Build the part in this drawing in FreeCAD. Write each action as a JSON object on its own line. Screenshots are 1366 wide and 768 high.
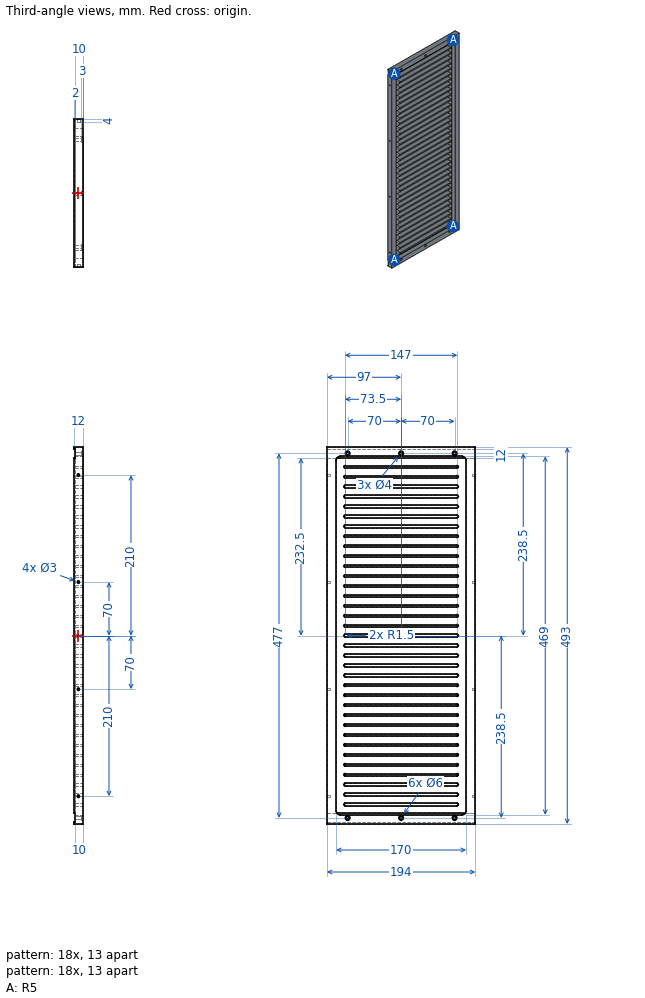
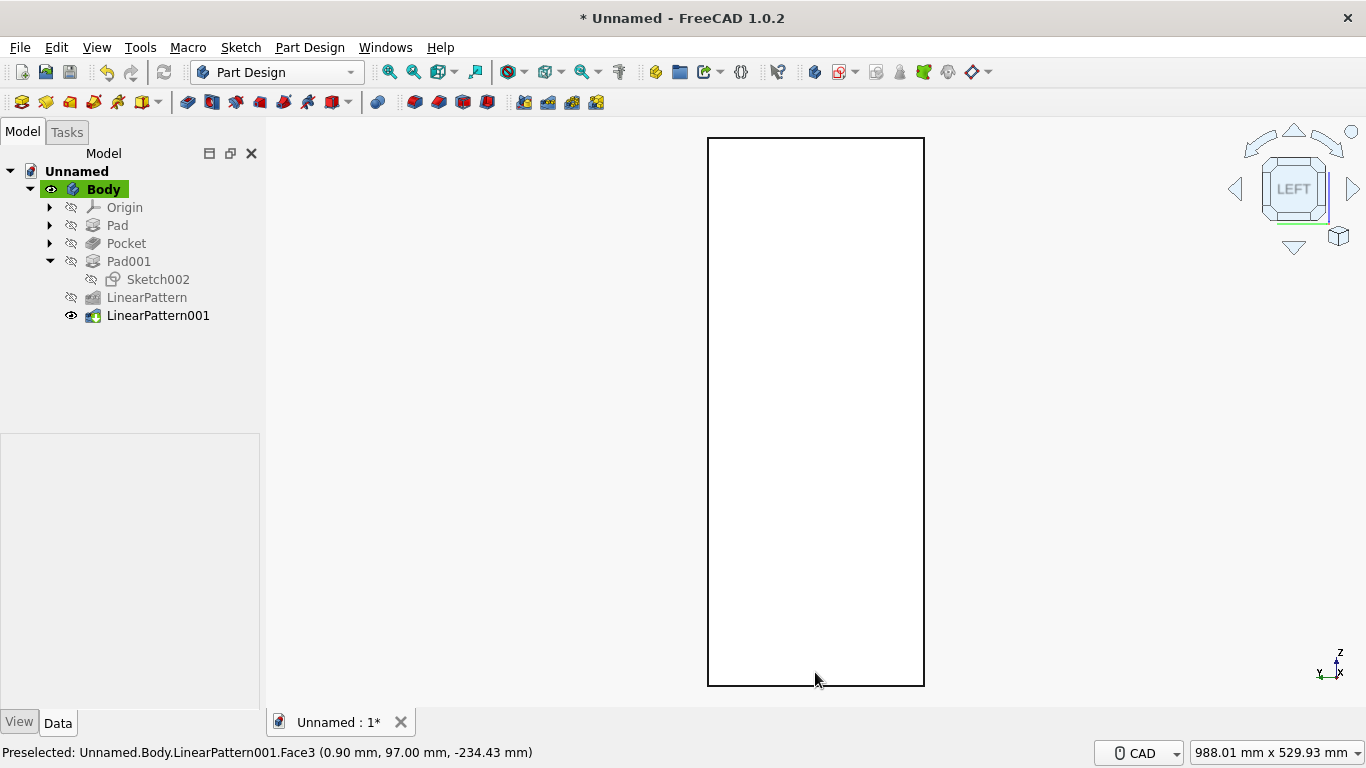
{"action": "scroll", "coordinate": [911, 672], "scroll_direction": "up", "scroll_amount": 7}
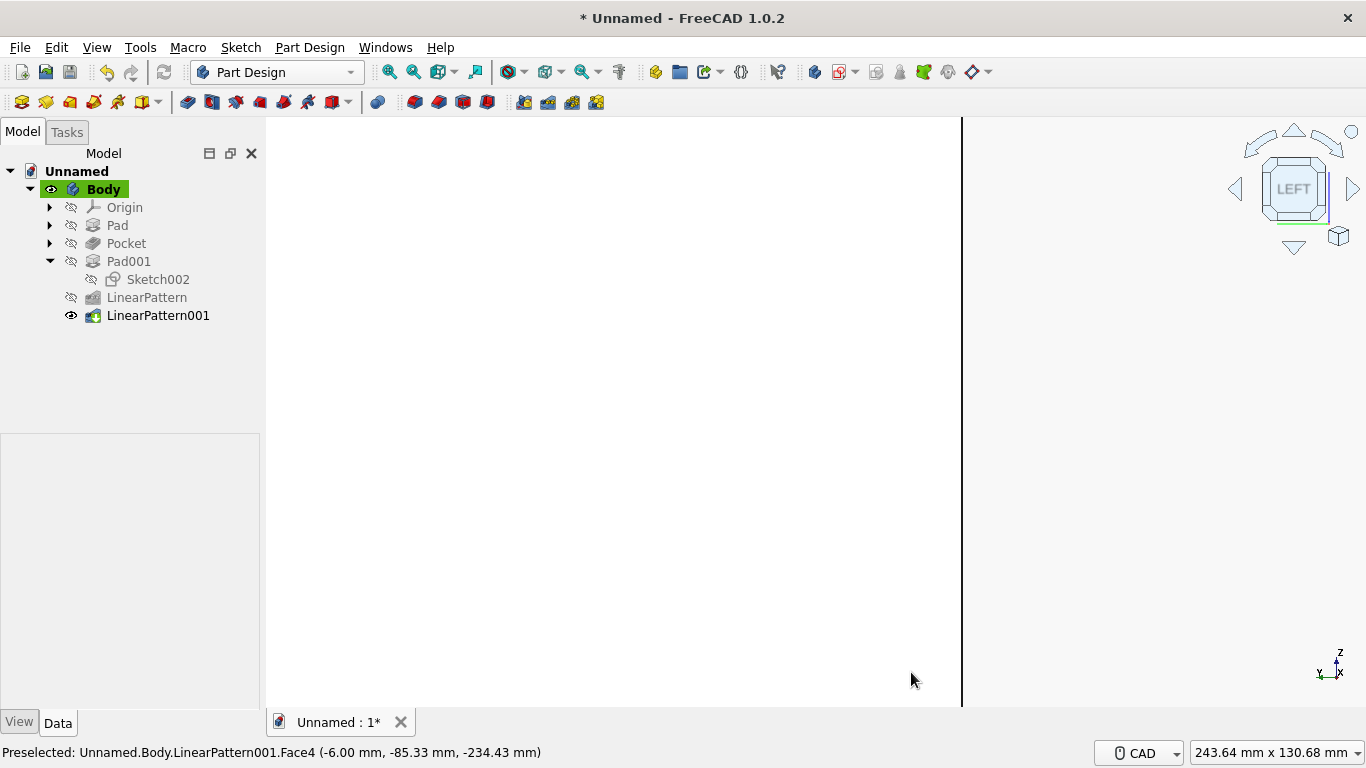
{"action": "key", "text": "v f"}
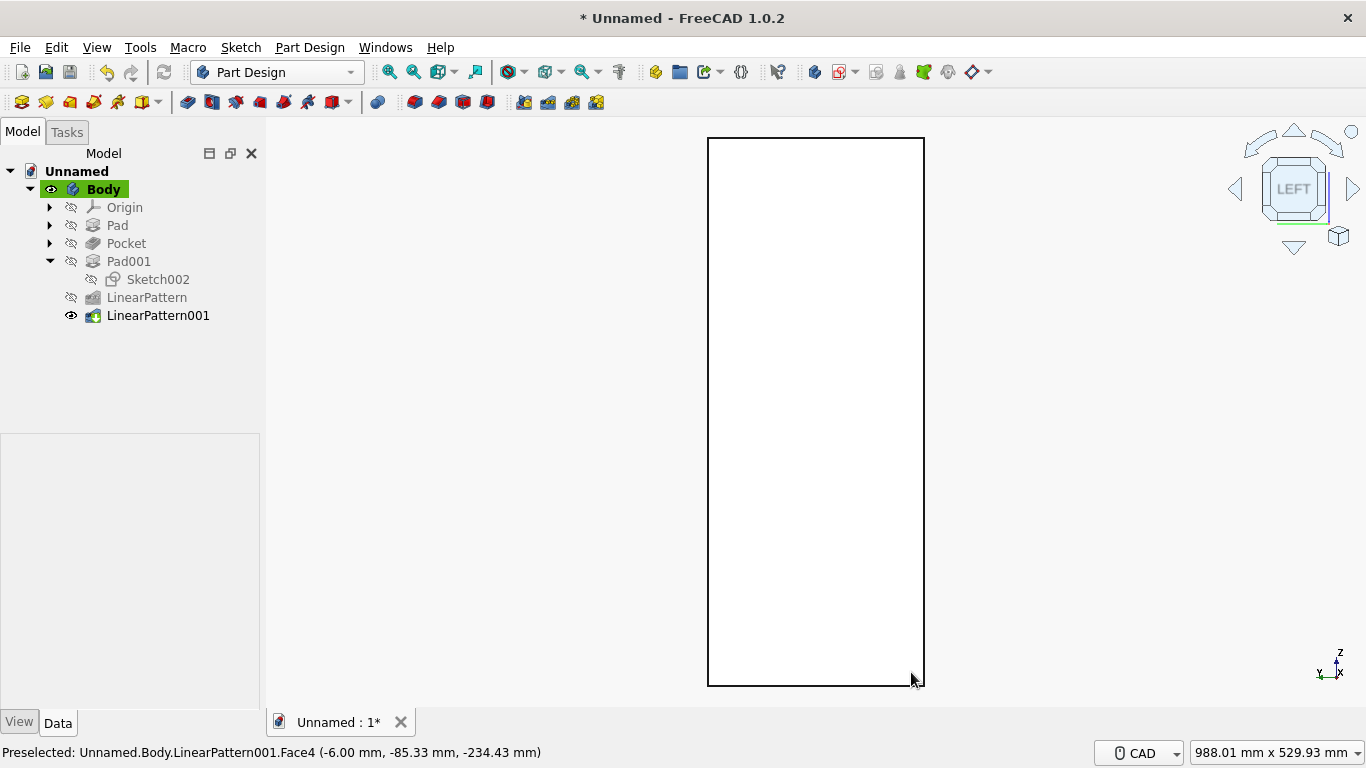
{"action": "key", "text": "v 3"}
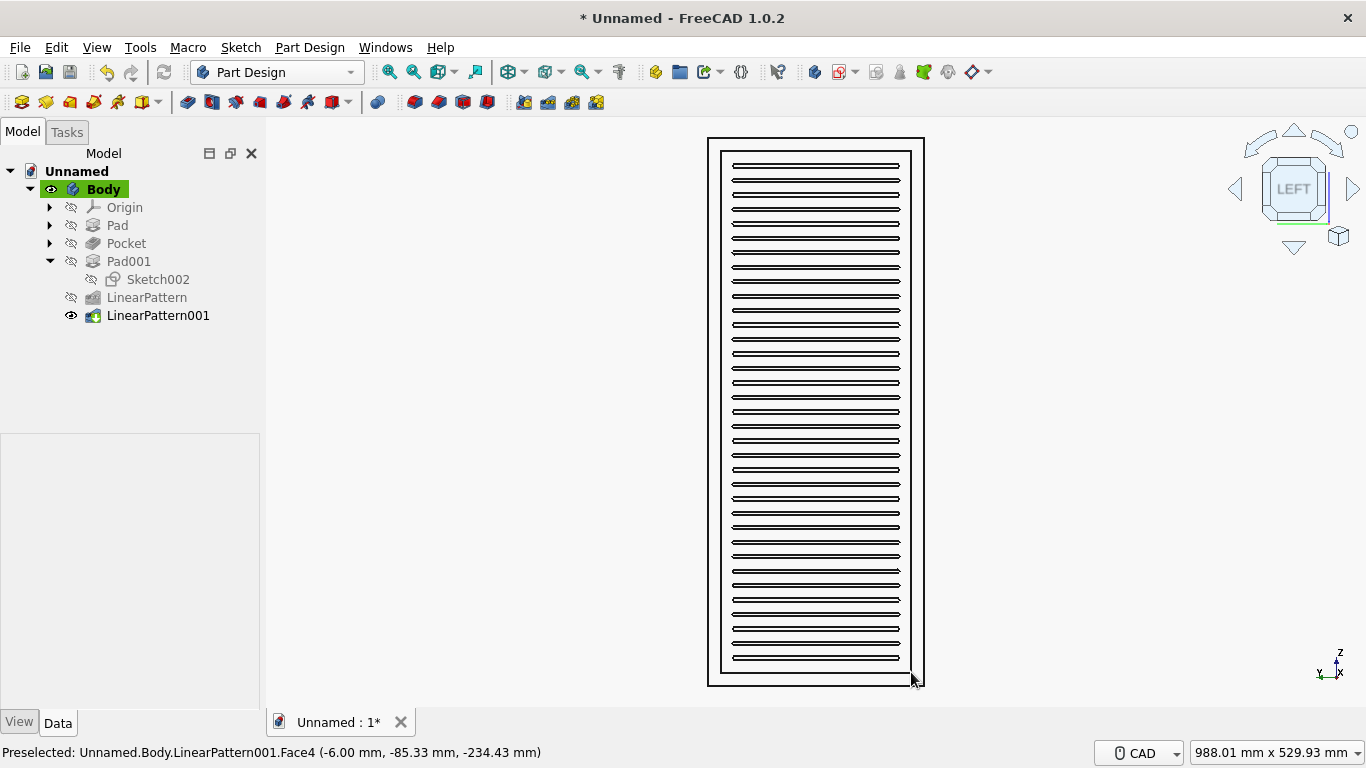
{"action": "key", "text": "0"}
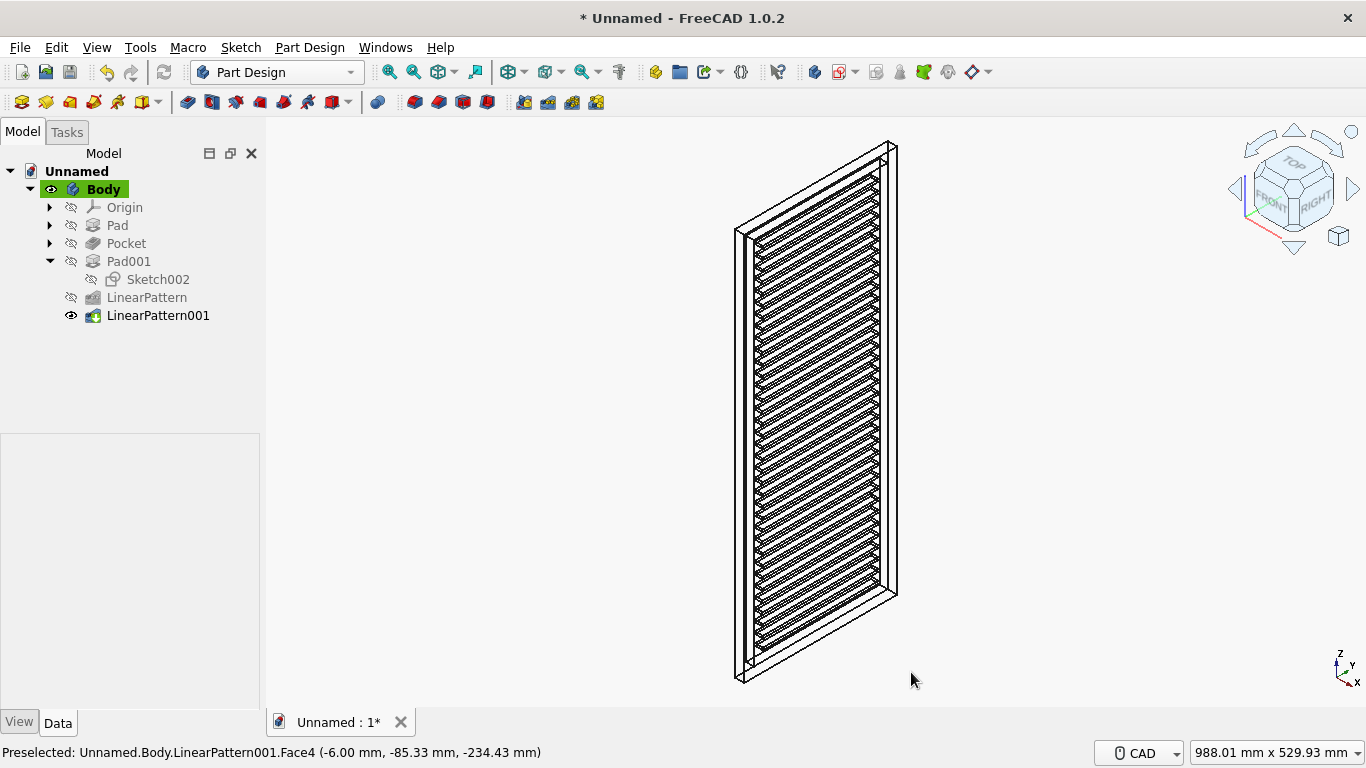
{"action": "scroll", "coordinate": [750, 663], "scroll_direction": "up", "scroll_amount": 7}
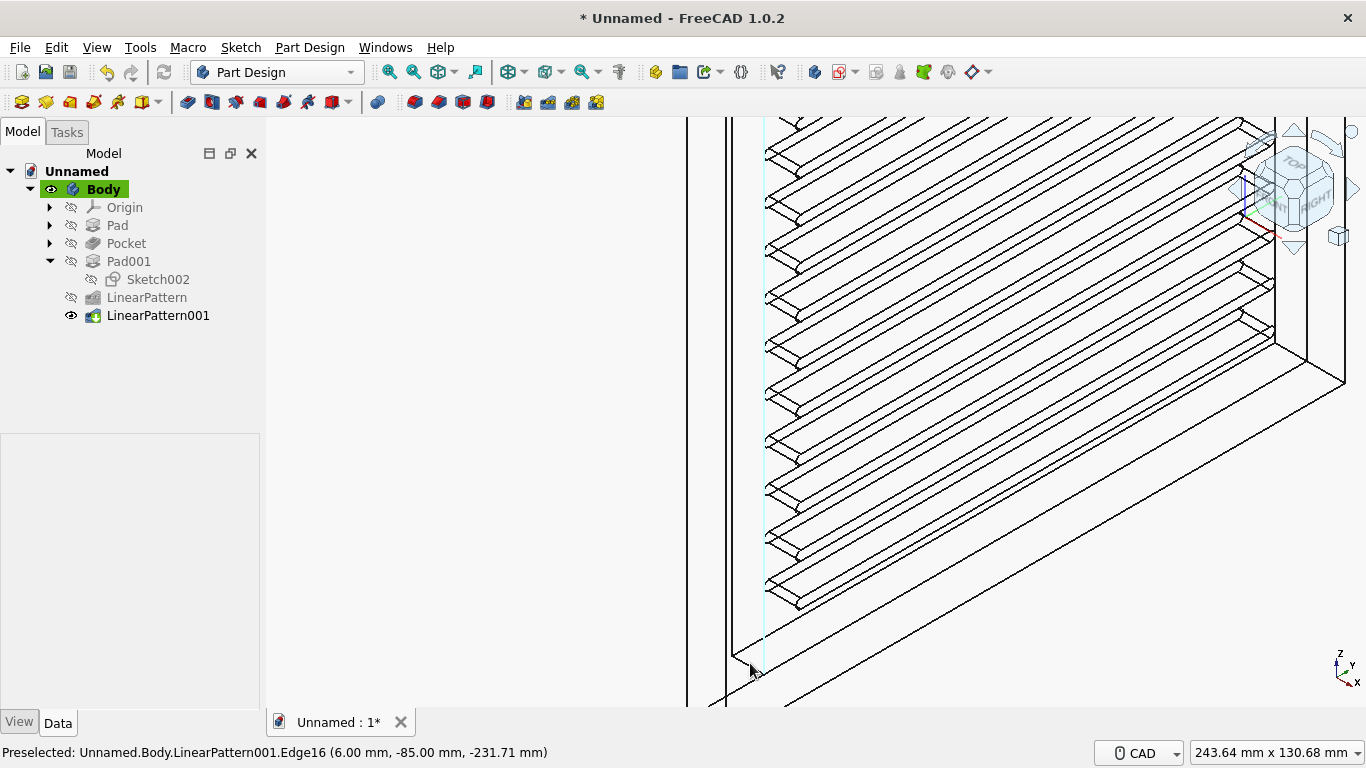
{"action": "left_click", "coordinate": [748, 664]}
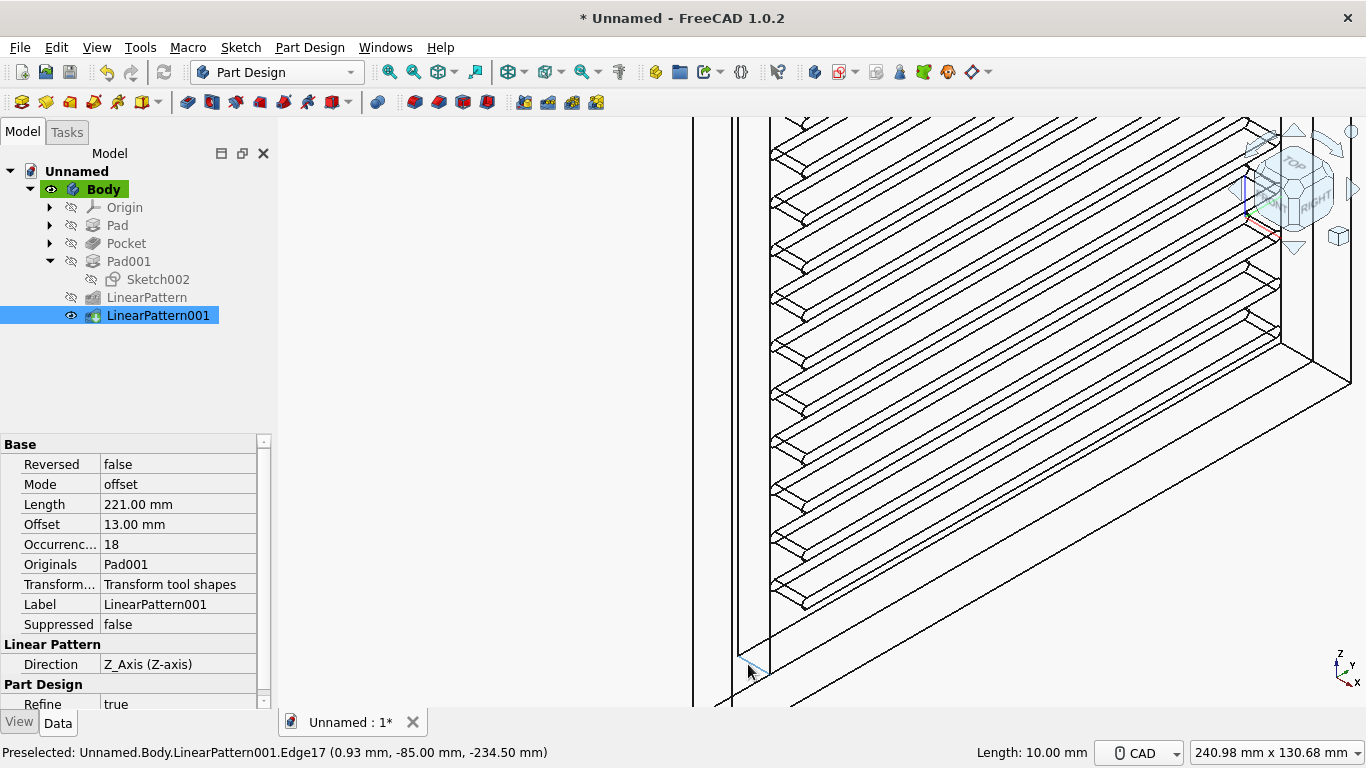
{"action": "left_click", "coordinate": [1297, 351], "text": "ctrl"}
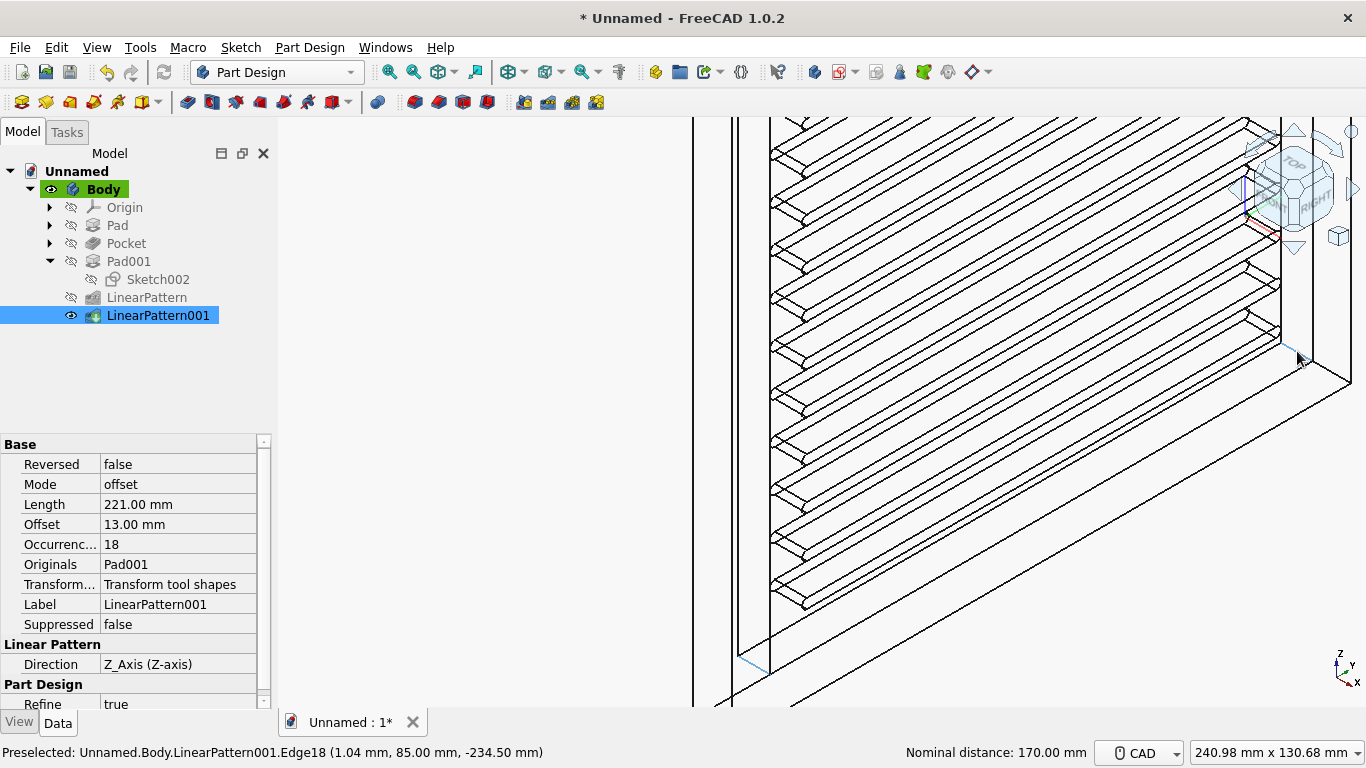
{"action": "key", "text": "v f"}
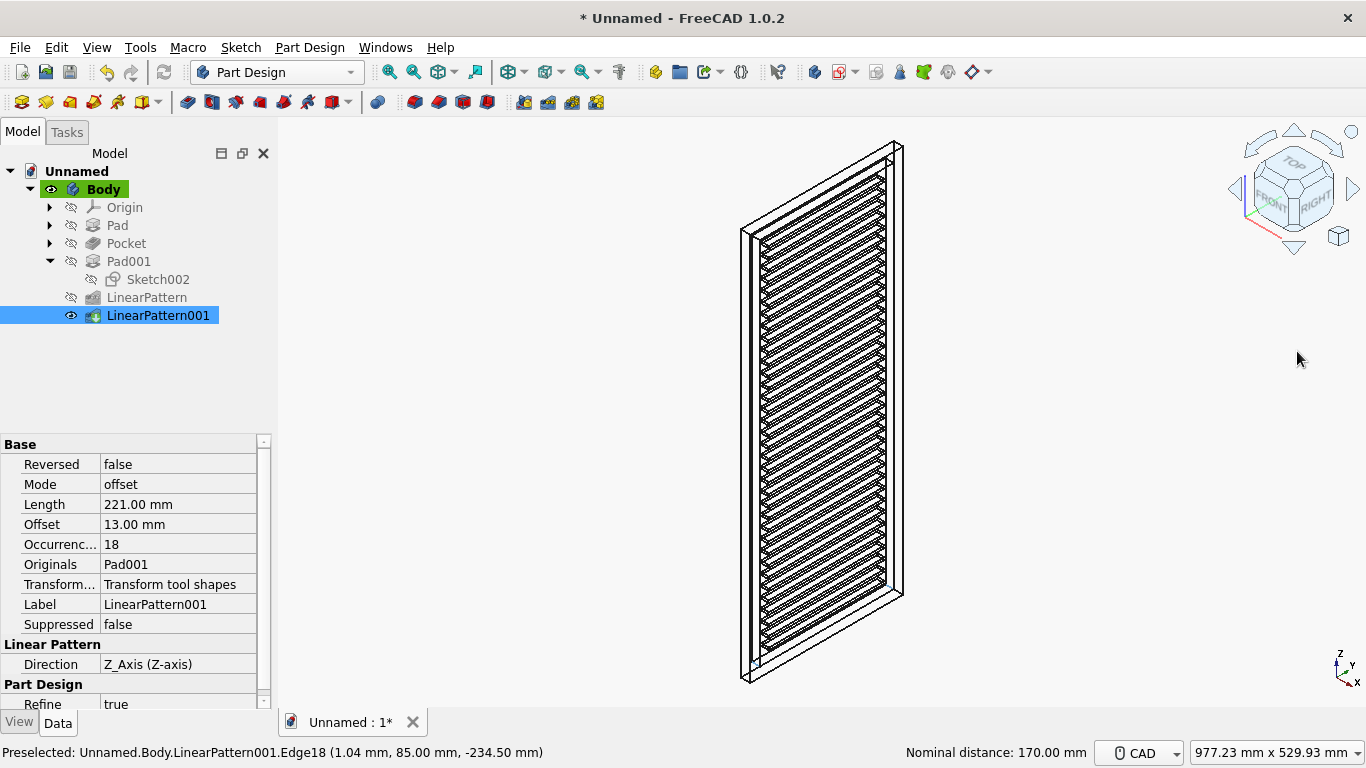
{"action": "key", "text": "2"}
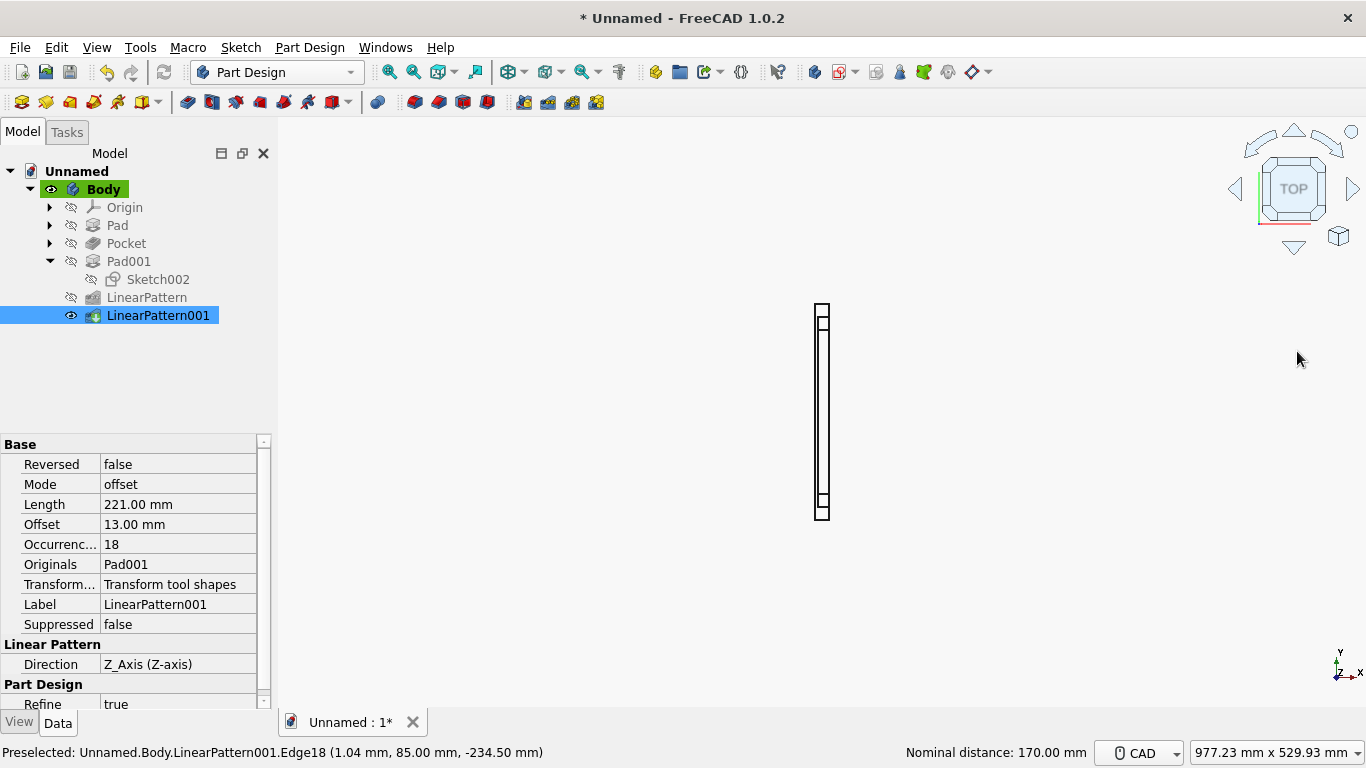
{"action": "left_click", "coordinate": [390, 72]}